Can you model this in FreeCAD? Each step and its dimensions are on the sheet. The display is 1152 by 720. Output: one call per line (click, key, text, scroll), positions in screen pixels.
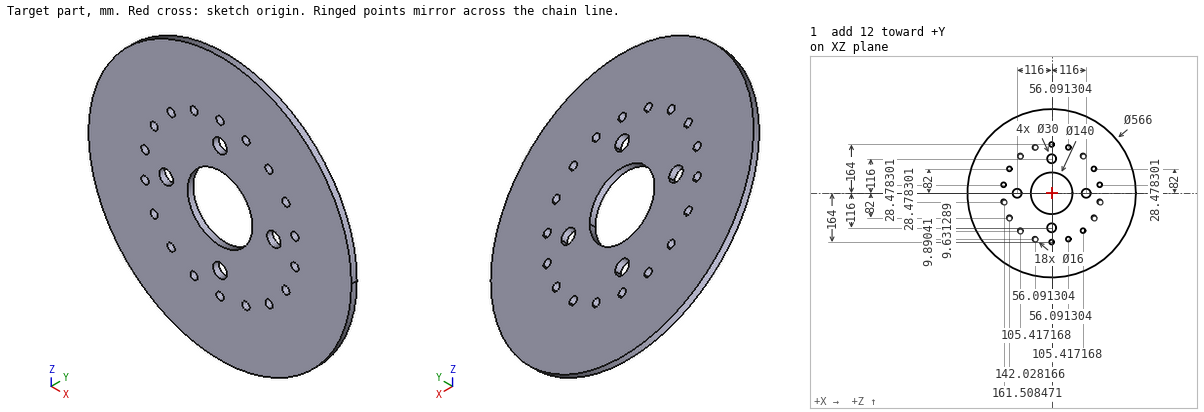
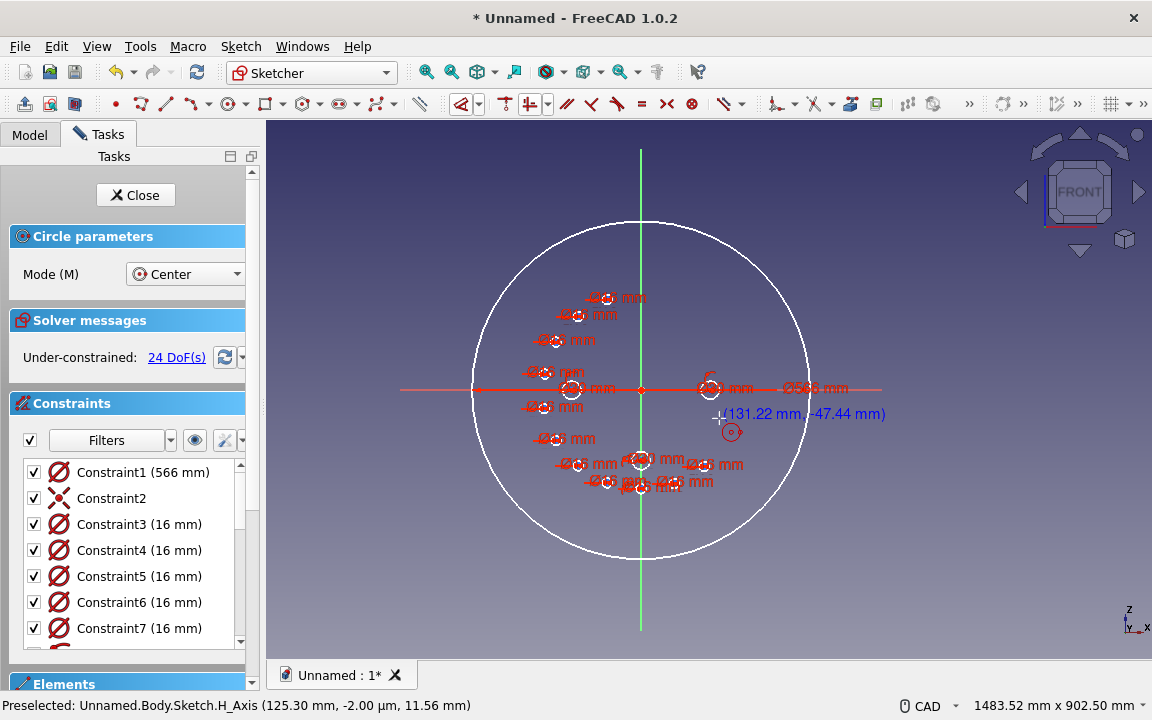
click(726, 439)
move(729, 436)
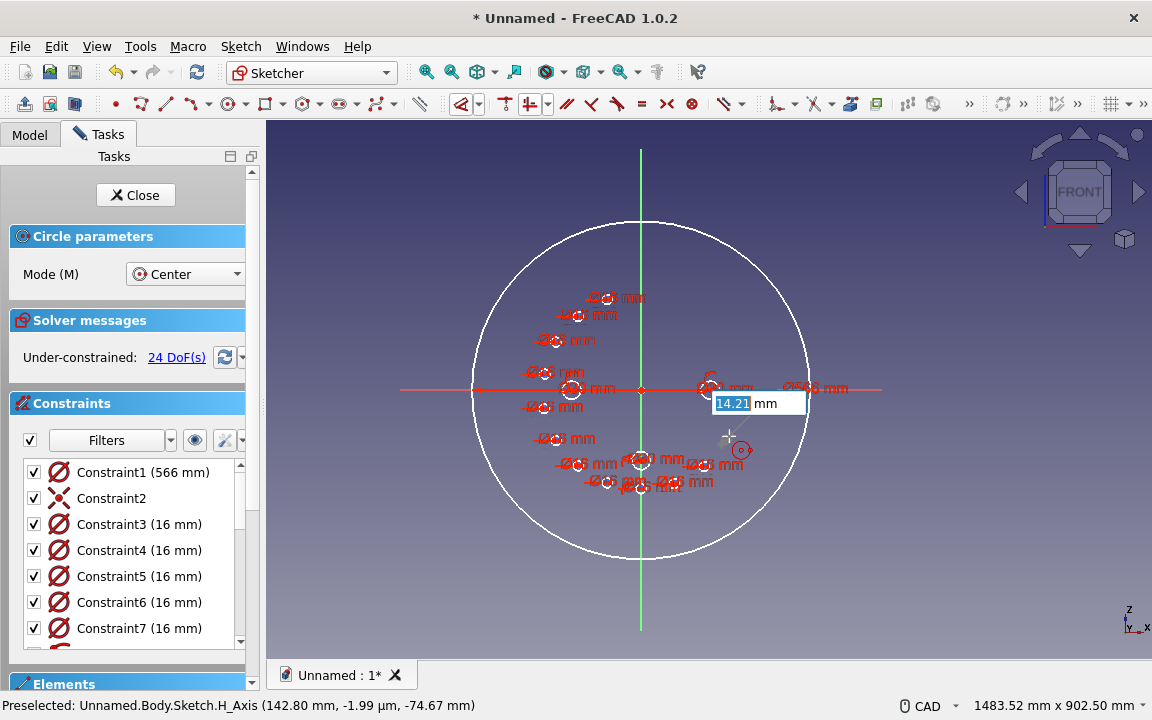
text(16)
key(Return)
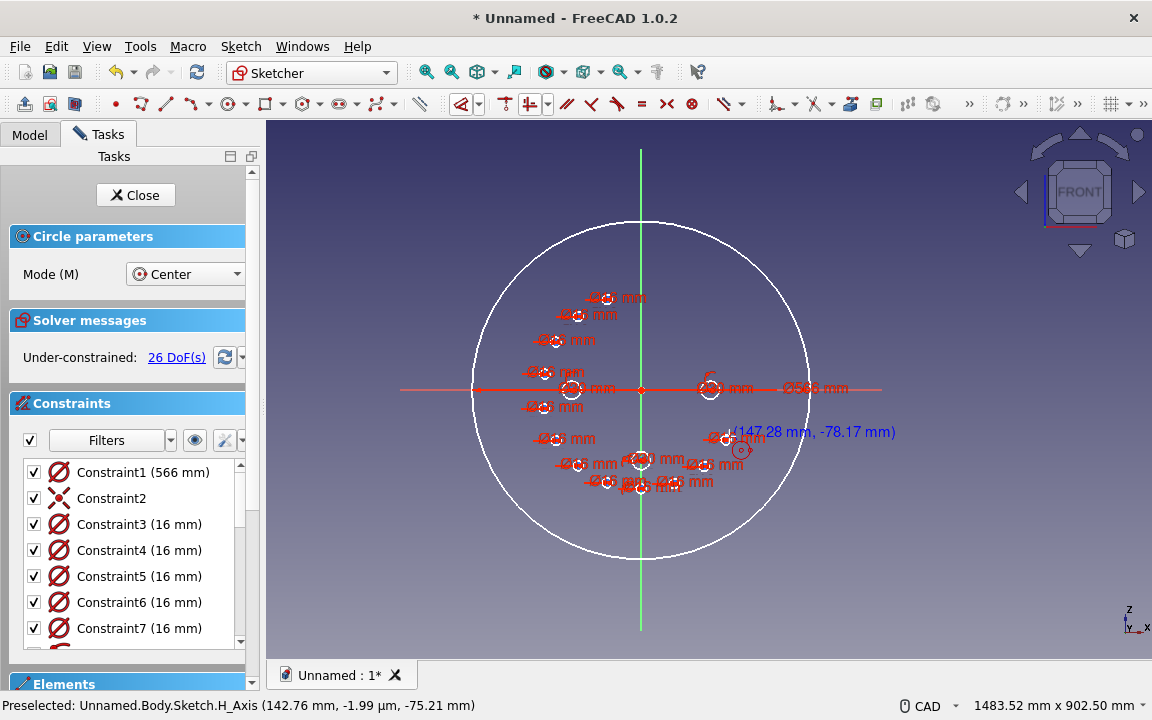
scroll(737, 407, up, 8)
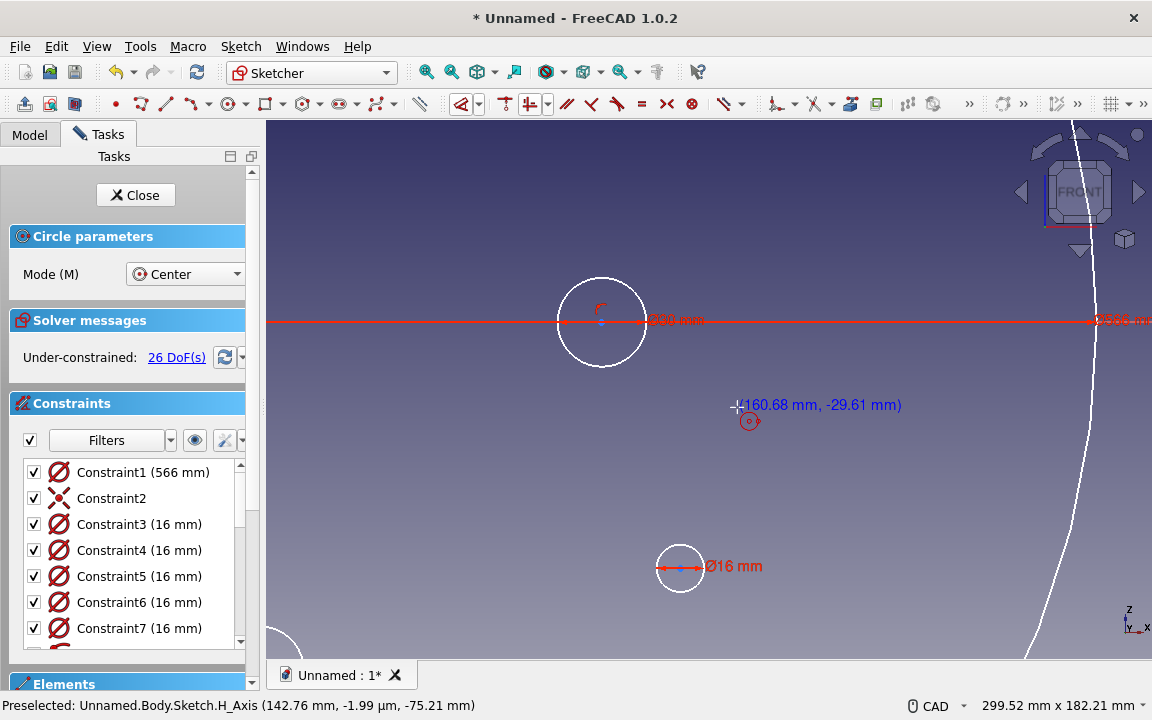
scroll(737, 407, down, 8)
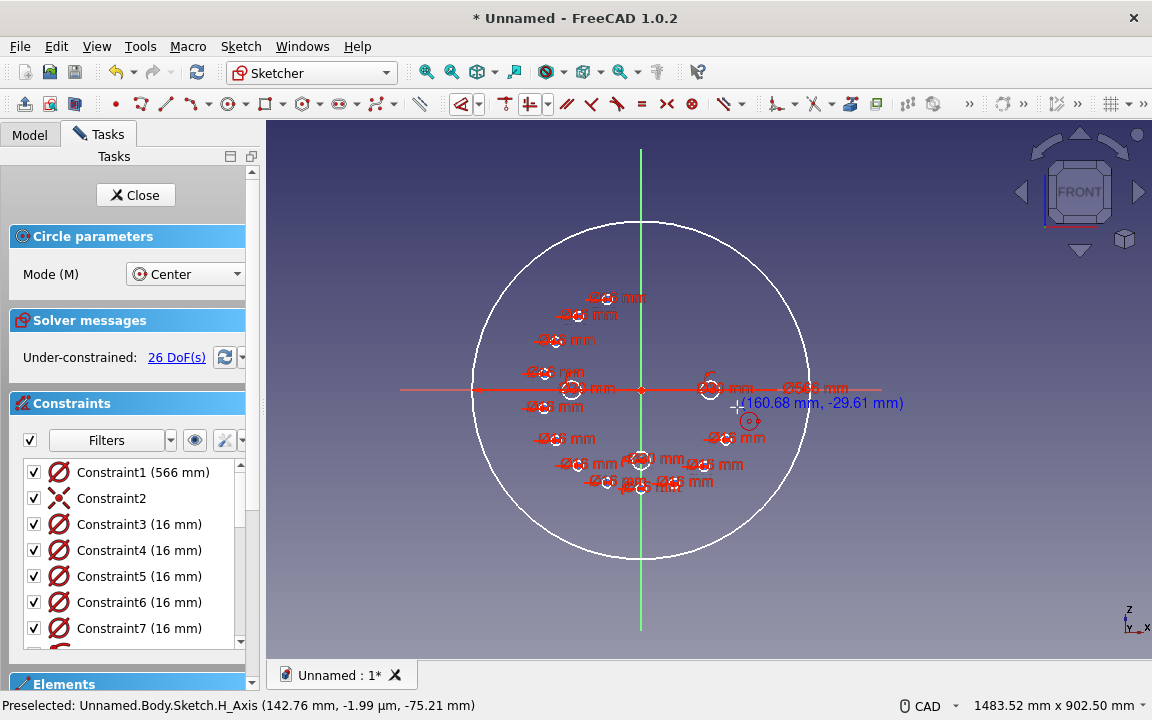
click(737, 407)
move(741, 411)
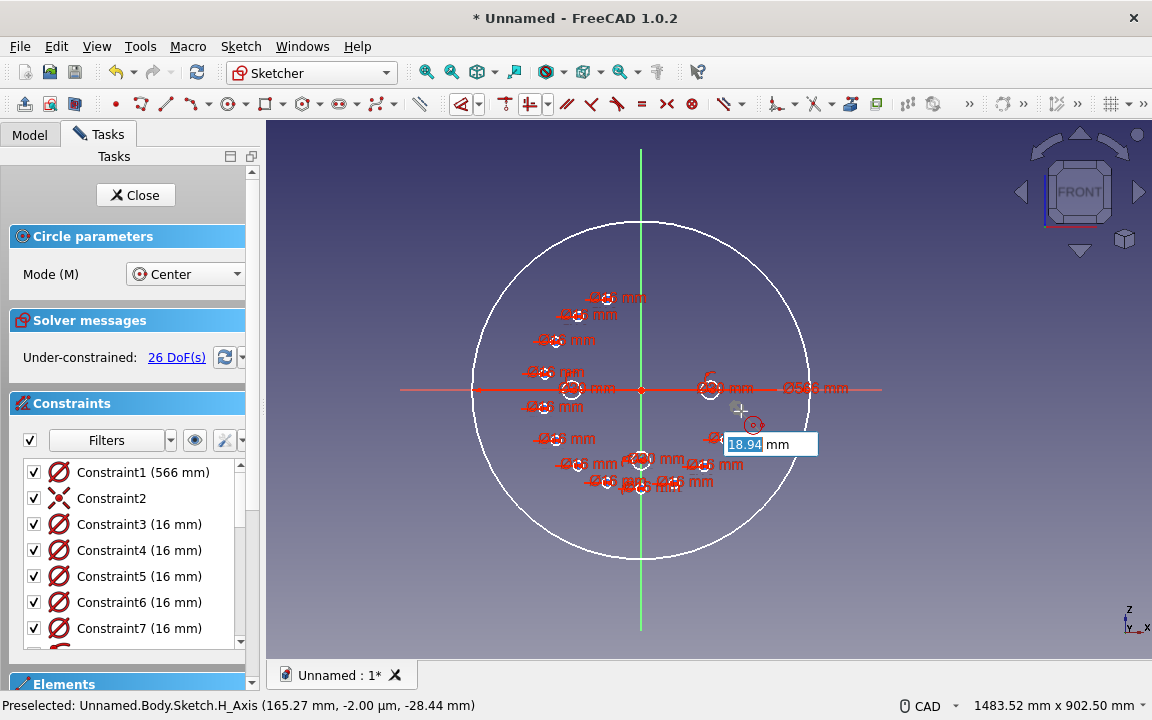
text(16)
key(Return)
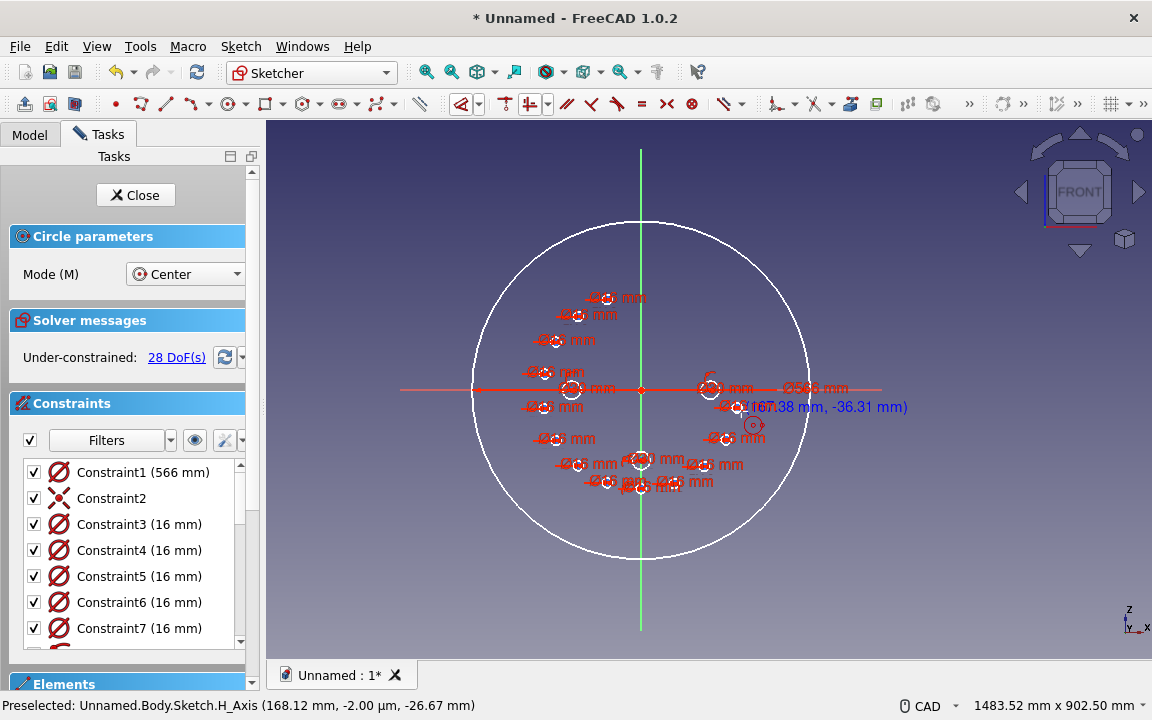
click(641, 390)
move(671, 361)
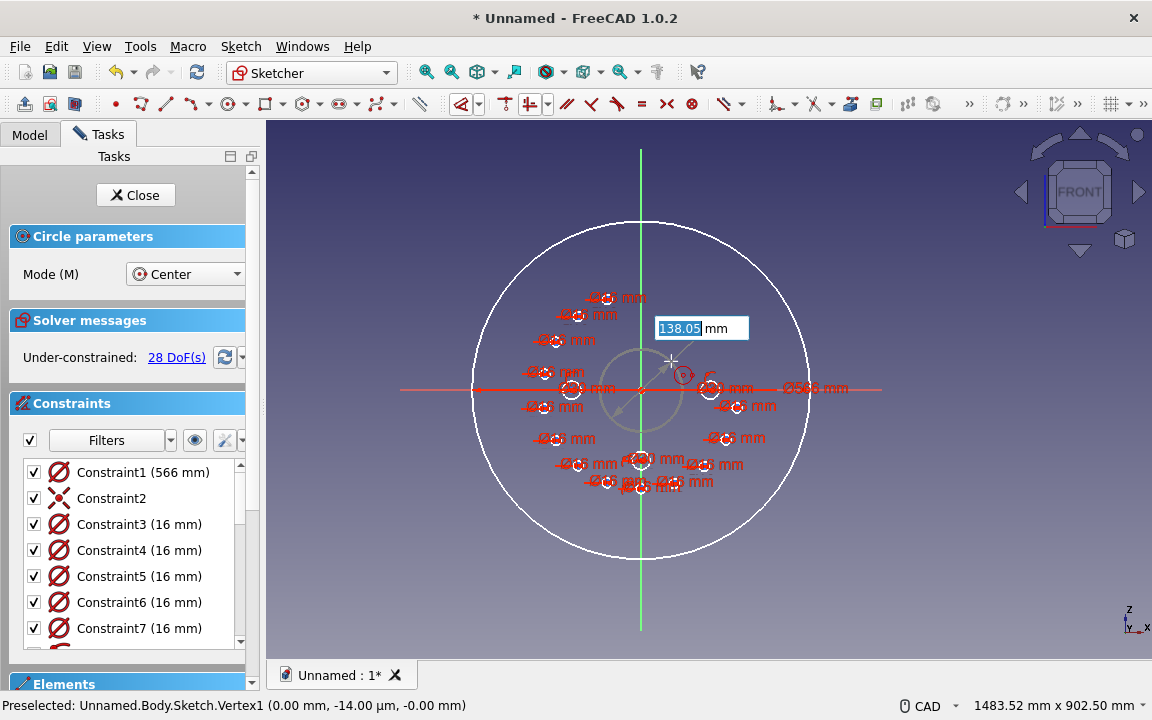
text(140)
key(Return)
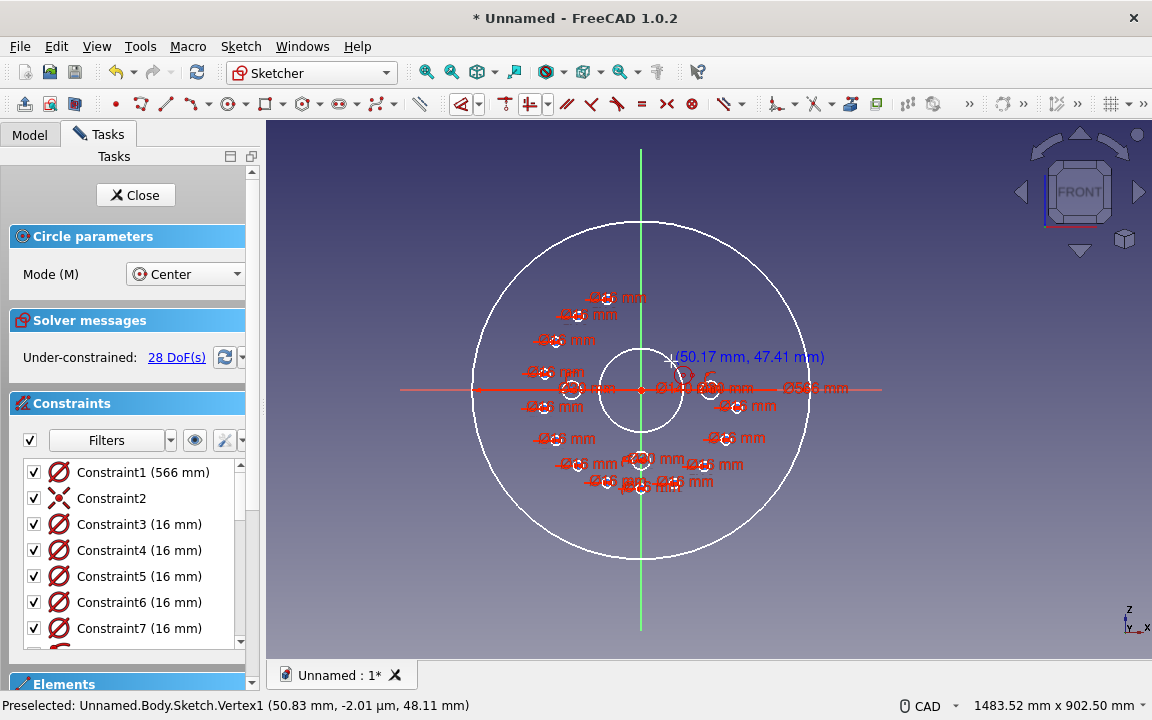
scroll(641, 321, up, 5)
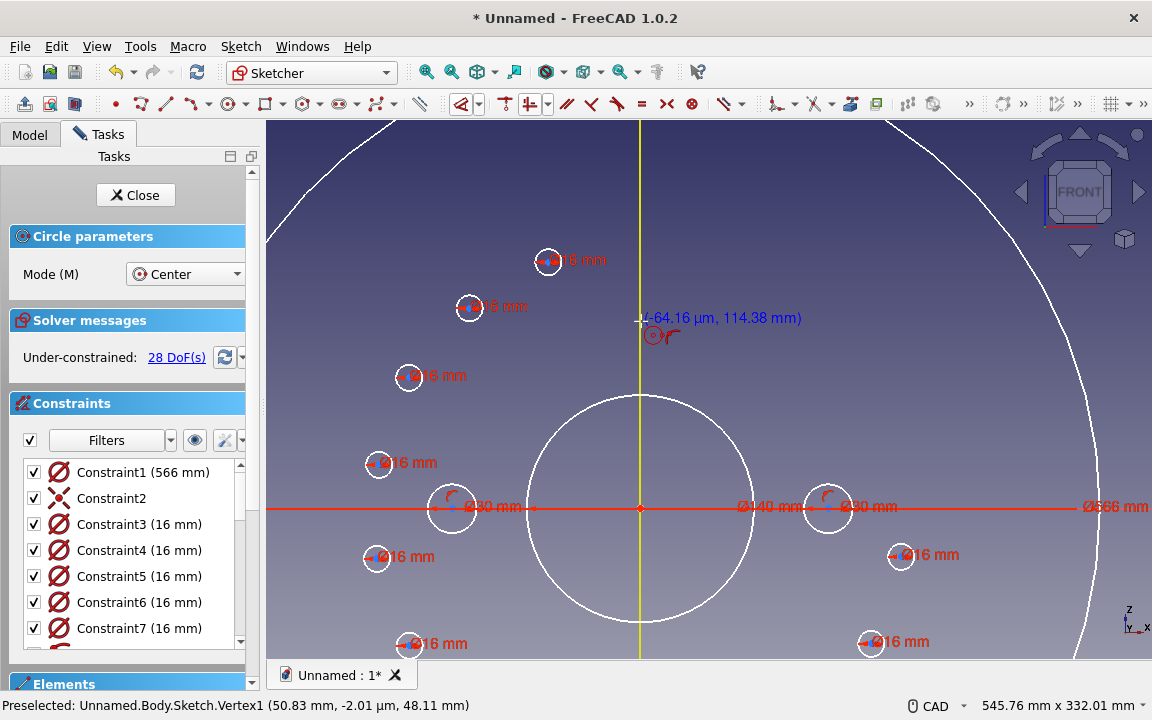
click(640, 320)
move(658, 303)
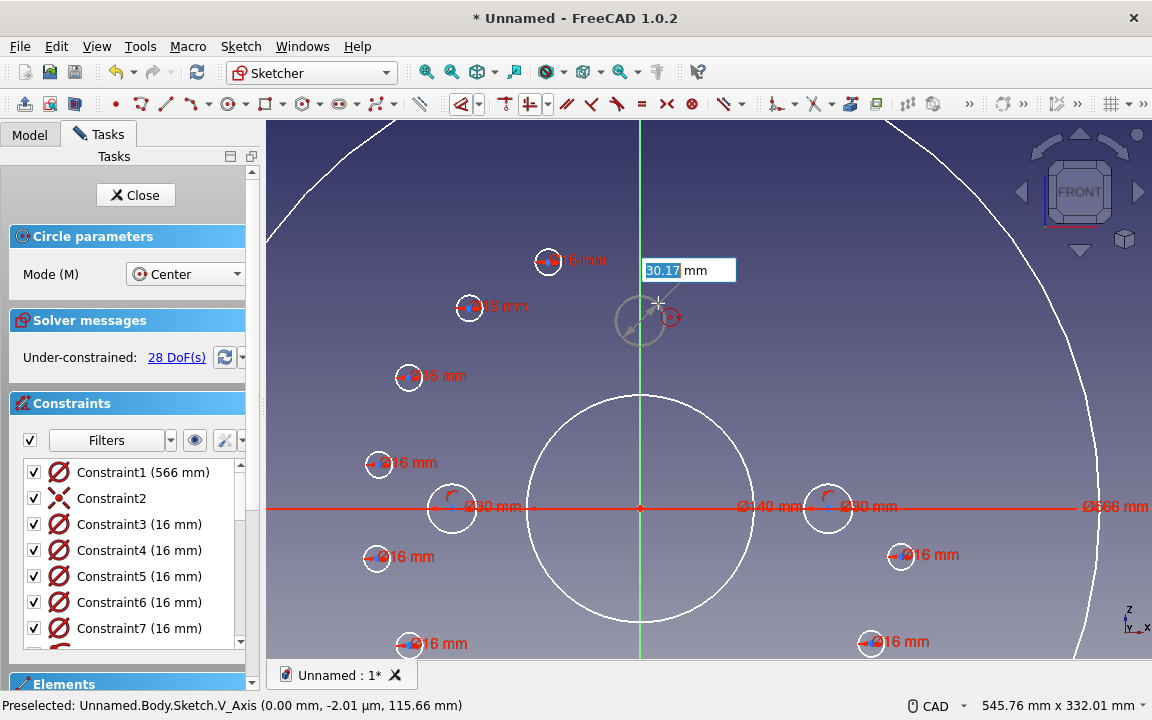
text(30)
key(Return)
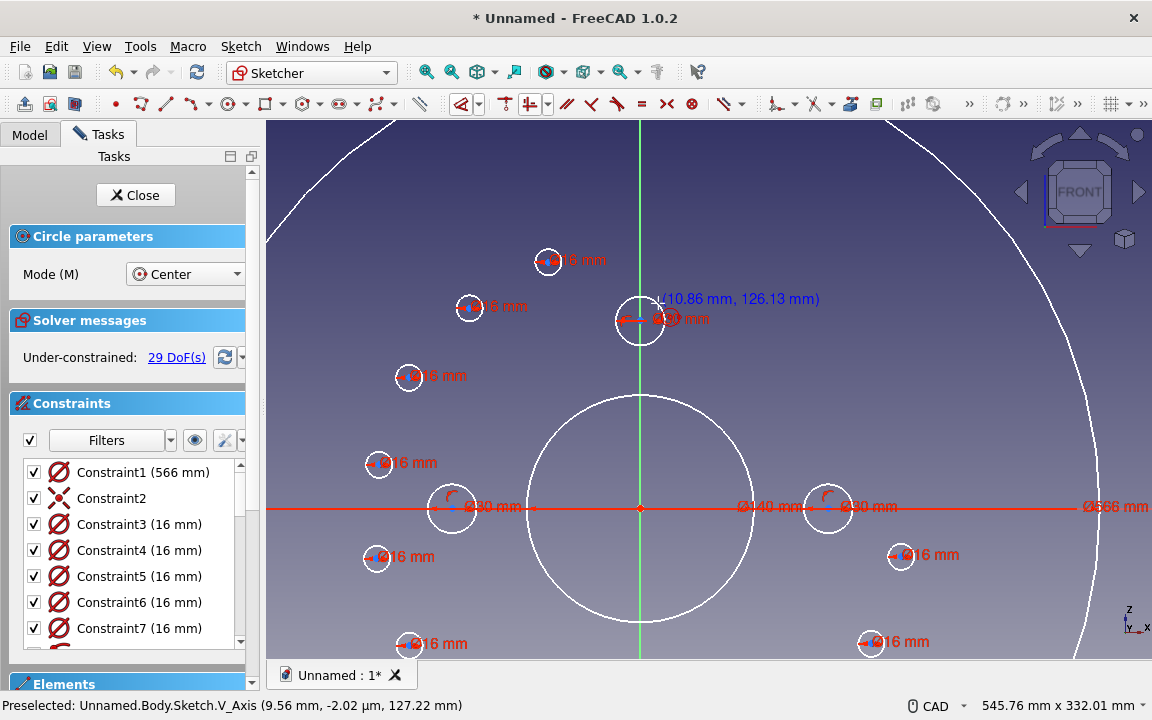
scroll(640, 243, up, 3)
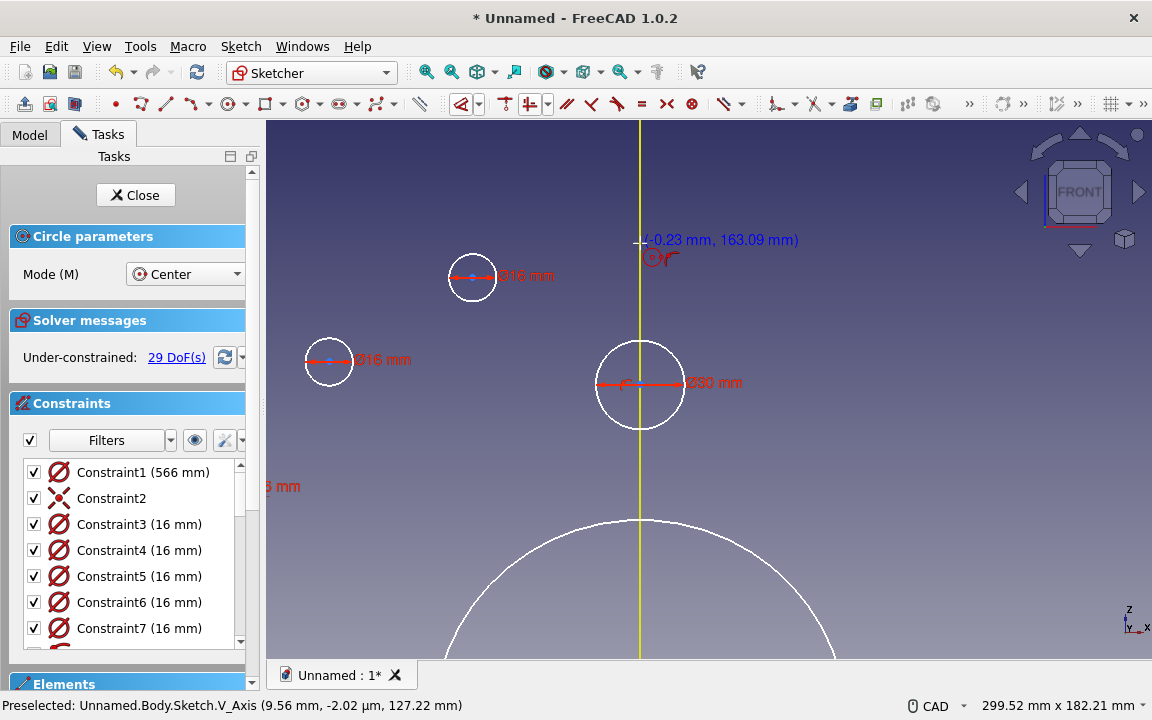
scroll(641, 304, down, 8)